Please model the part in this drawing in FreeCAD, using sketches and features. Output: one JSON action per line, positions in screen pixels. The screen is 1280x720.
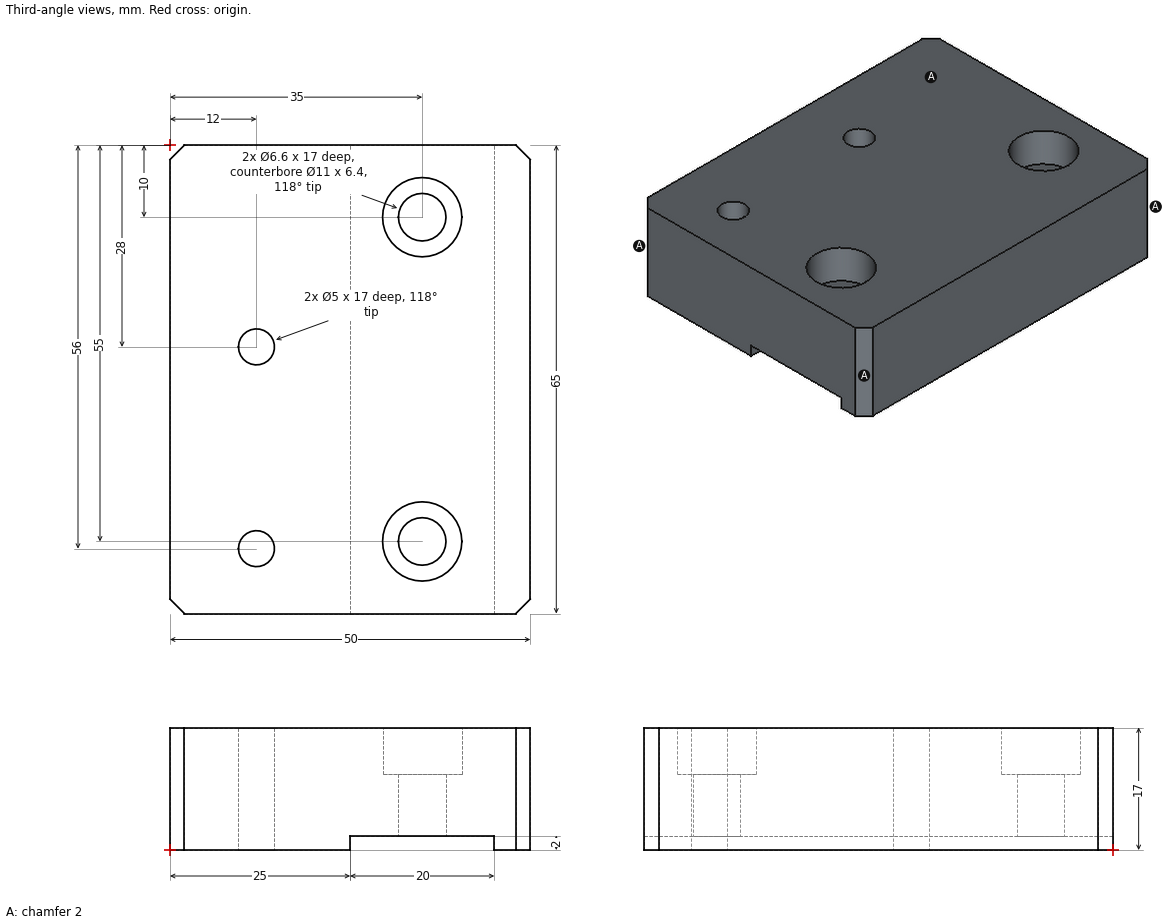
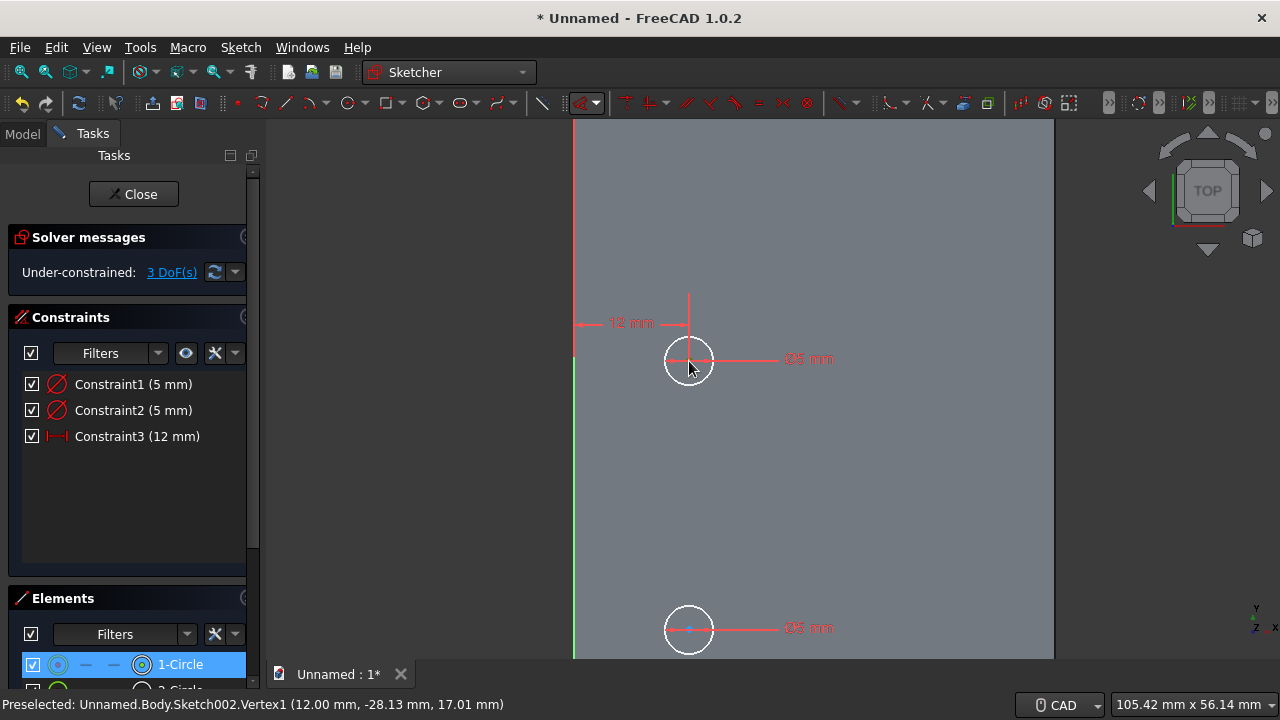
{"action": "key", "text": "i"}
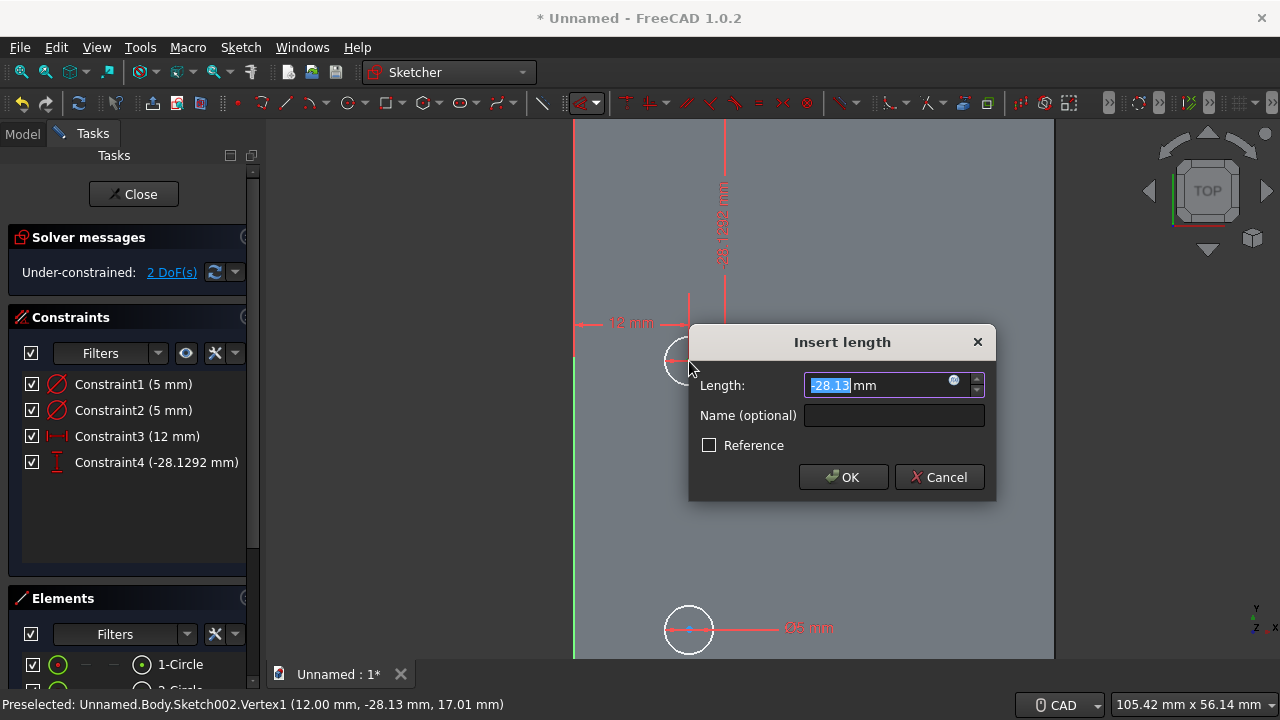
{"action": "type", "text": "-28"}
{"action": "key", "text": "Return"}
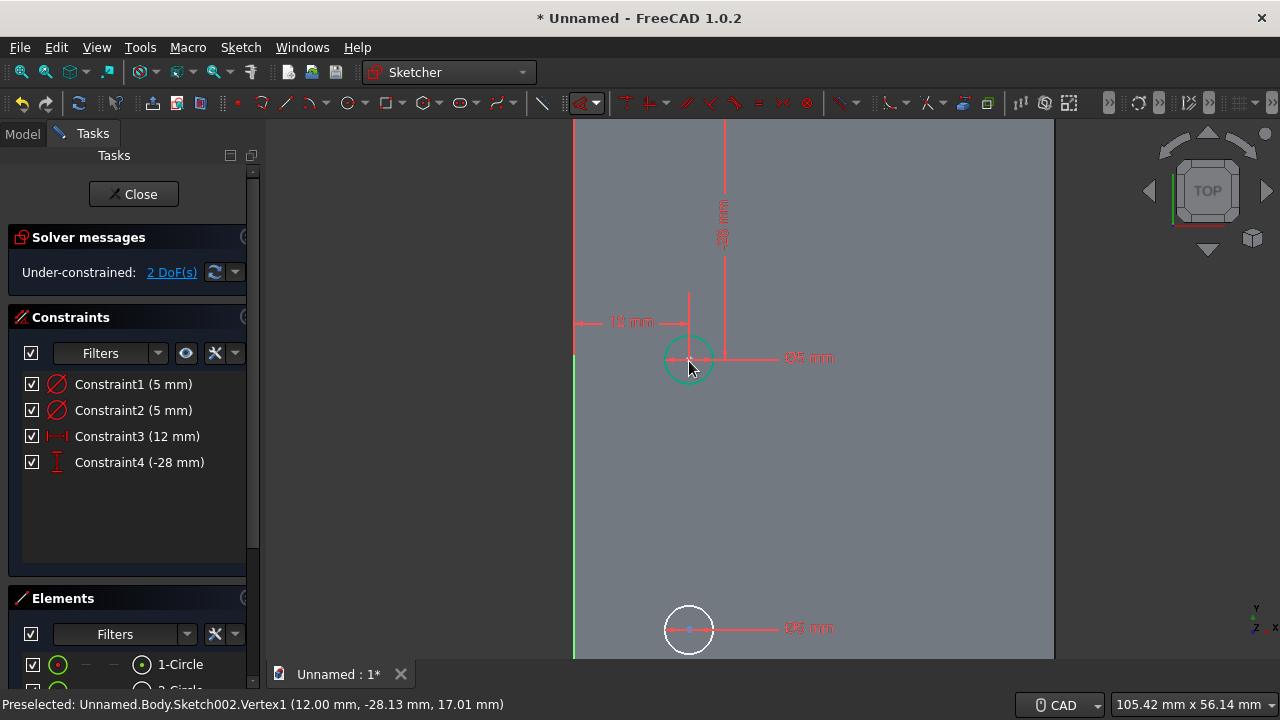
{"action": "left_click", "coordinate": [689, 630]}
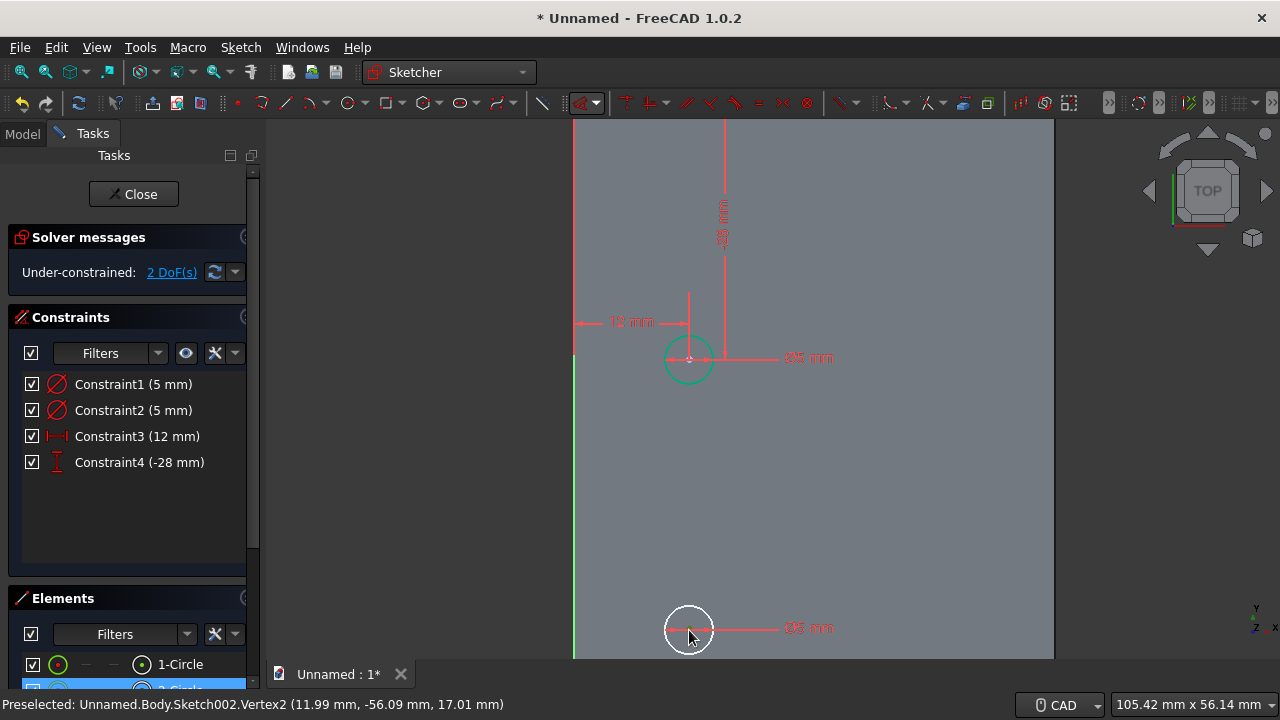
{"action": "left_click", "coordinate": [598, 104]}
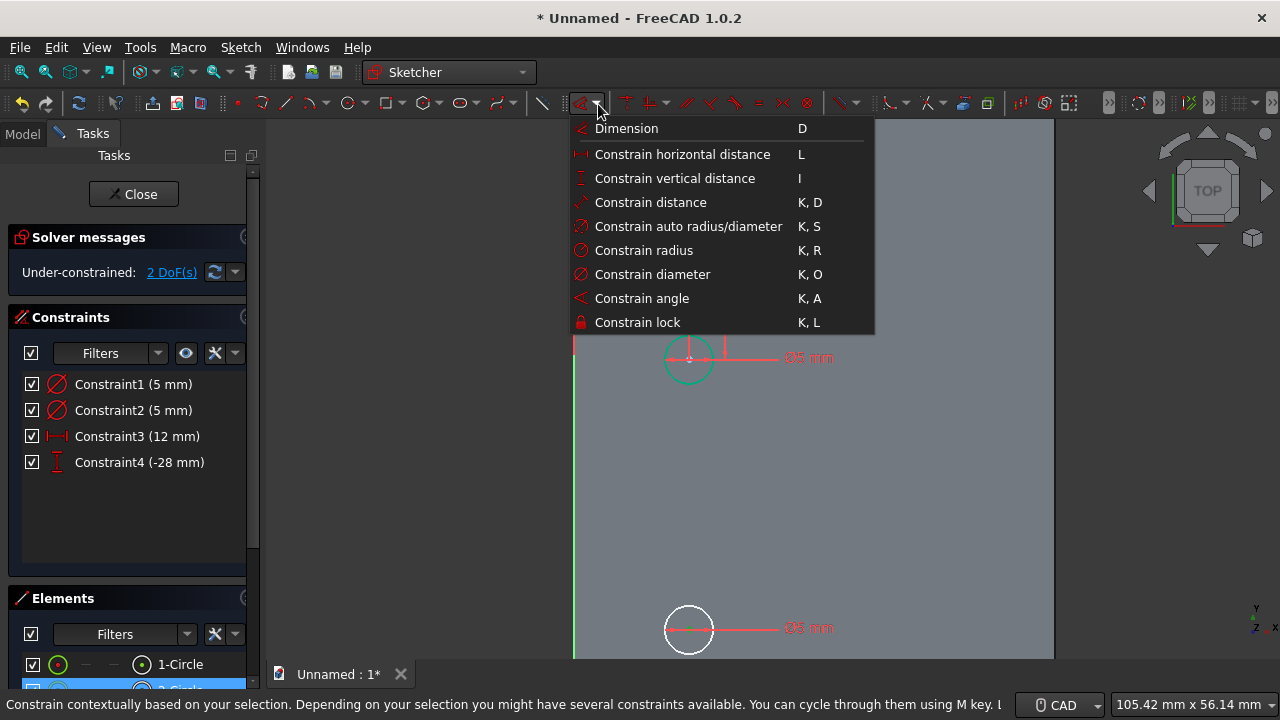
{"action": "left_click", "coordinate": [722, 154]}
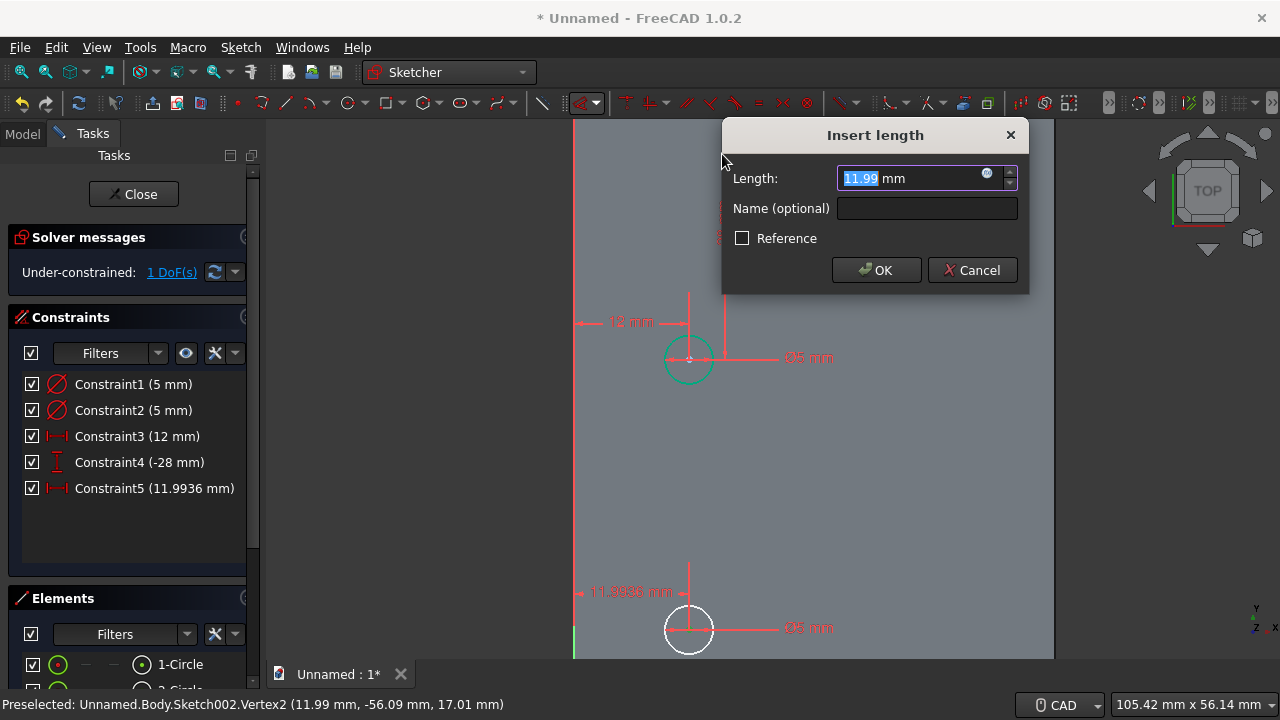
{"action": "type", "text": "12"}
{"action": "key", "text": "Return"}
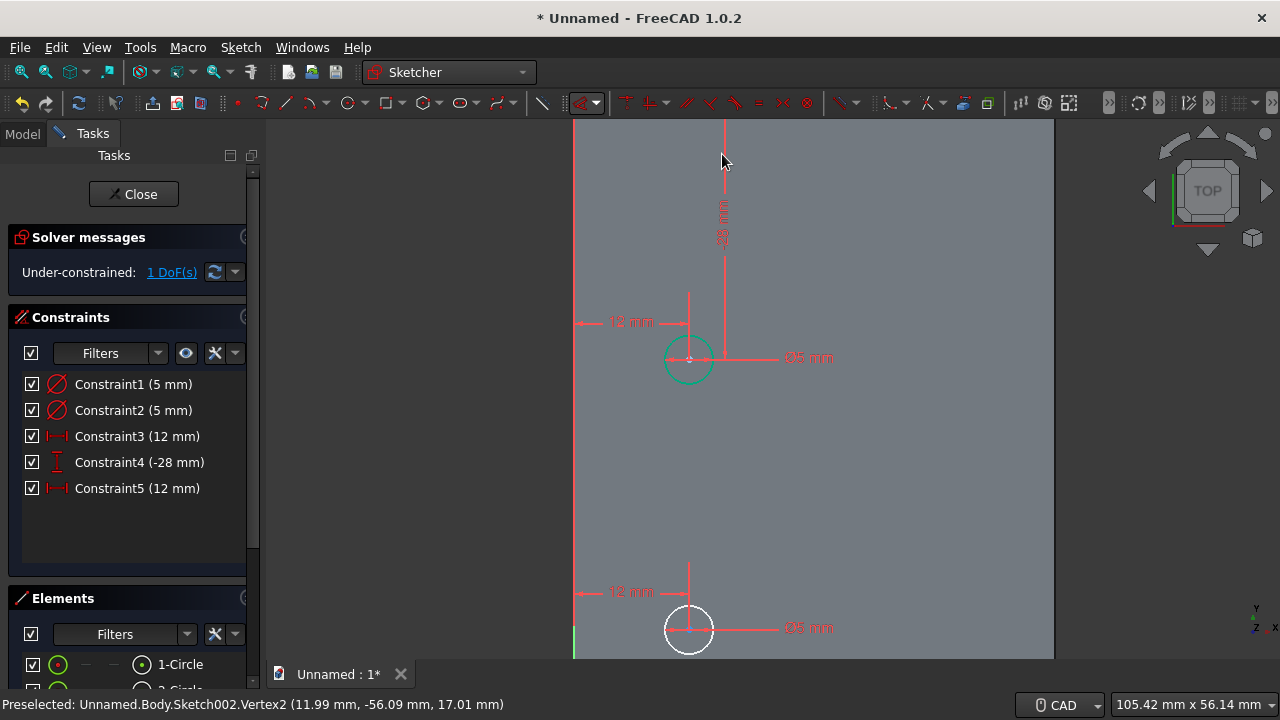
{"action": "left_click", "coordinate": [689, 630]}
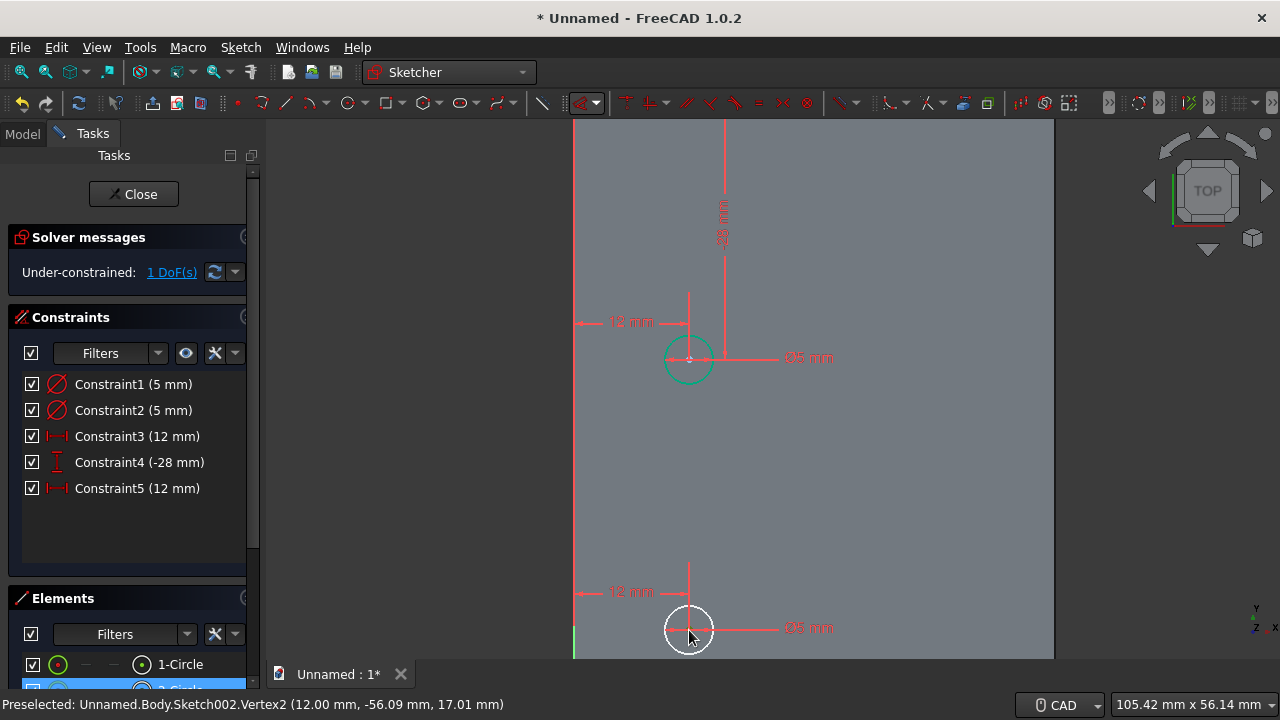
{"action": "left_click", "coordinate": [598, 104]}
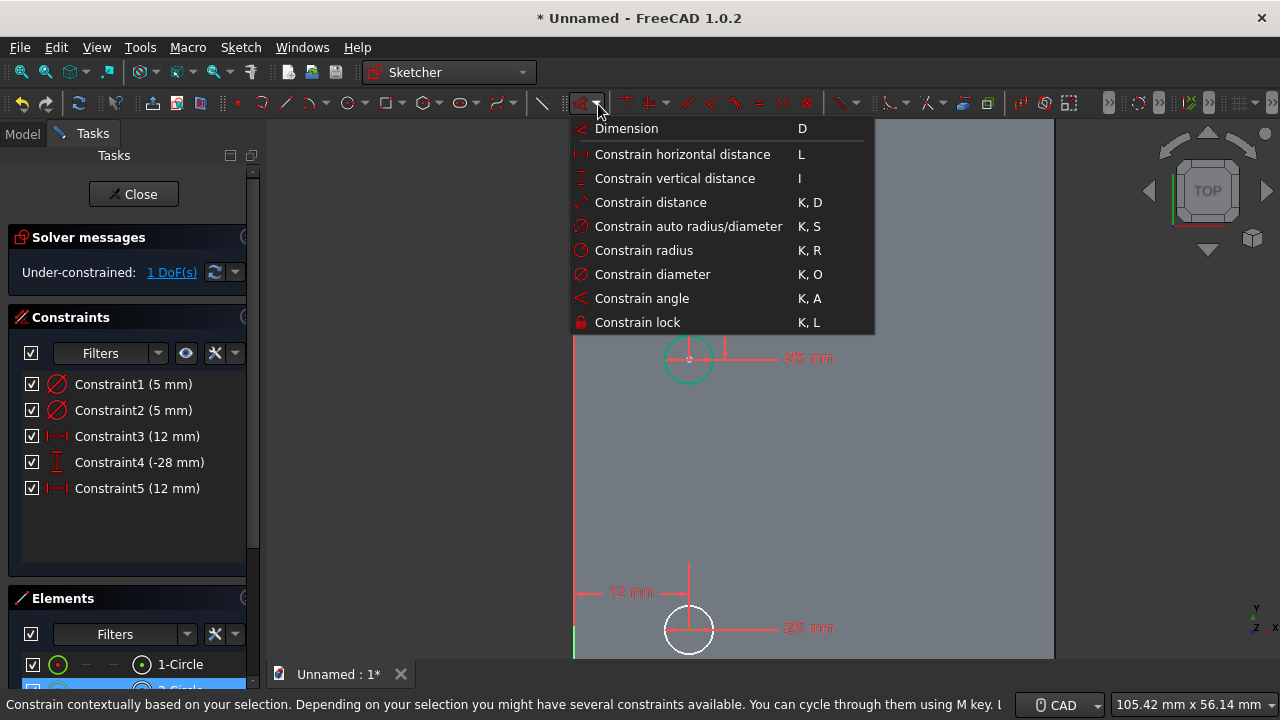
{"action": "left_click", "coordinate": [722, 178]}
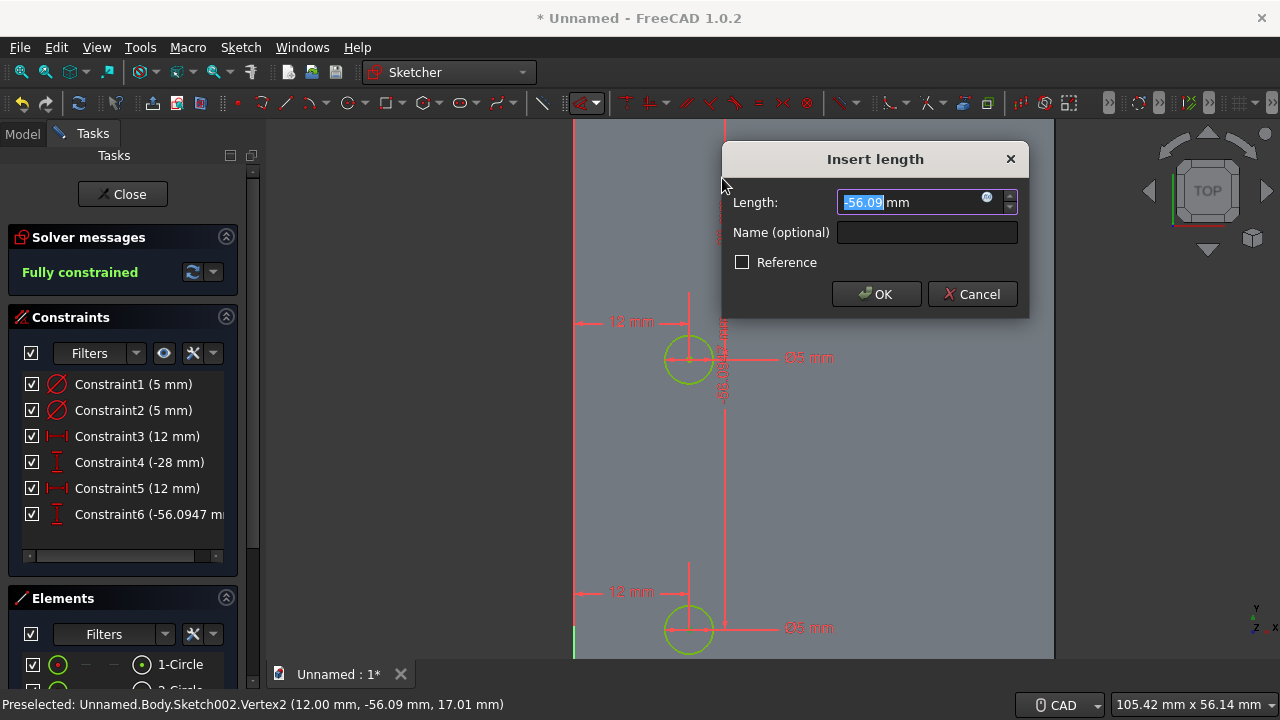
{"action": "type", "text": "-56"}
{"action": "key", "text": "Return"}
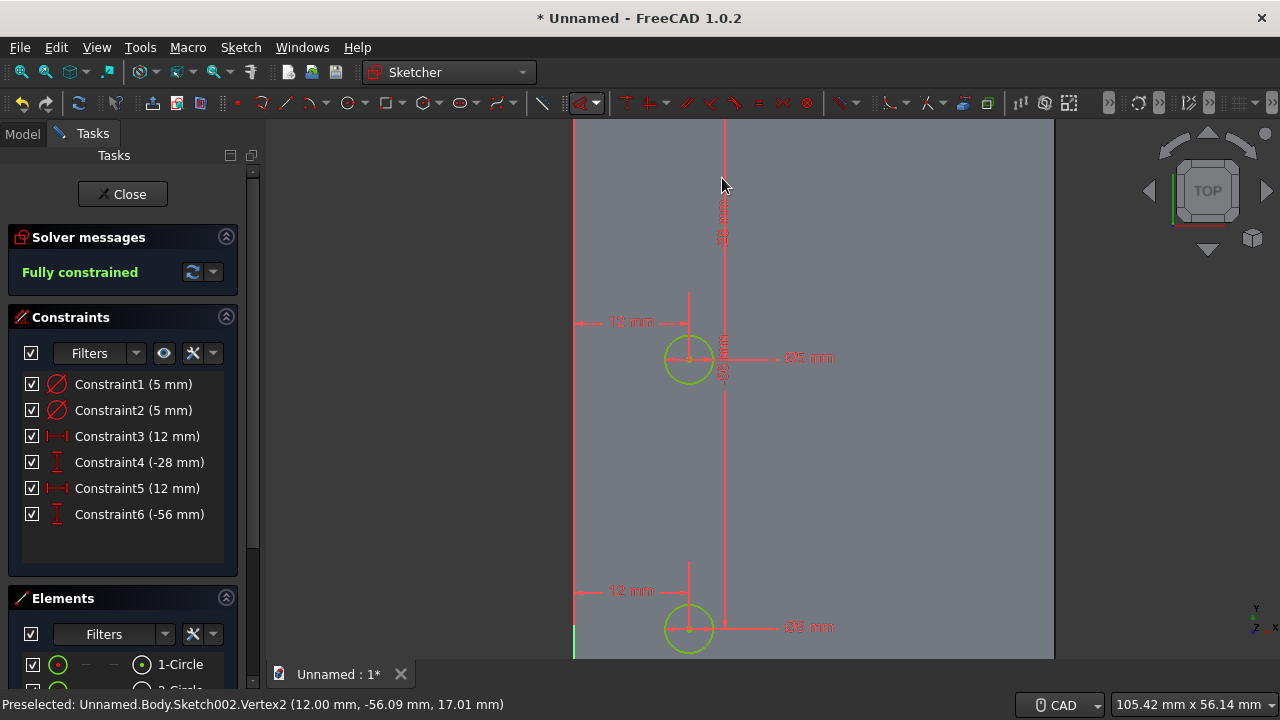
{"action": "left_click", "coordinate": [123, 194]}